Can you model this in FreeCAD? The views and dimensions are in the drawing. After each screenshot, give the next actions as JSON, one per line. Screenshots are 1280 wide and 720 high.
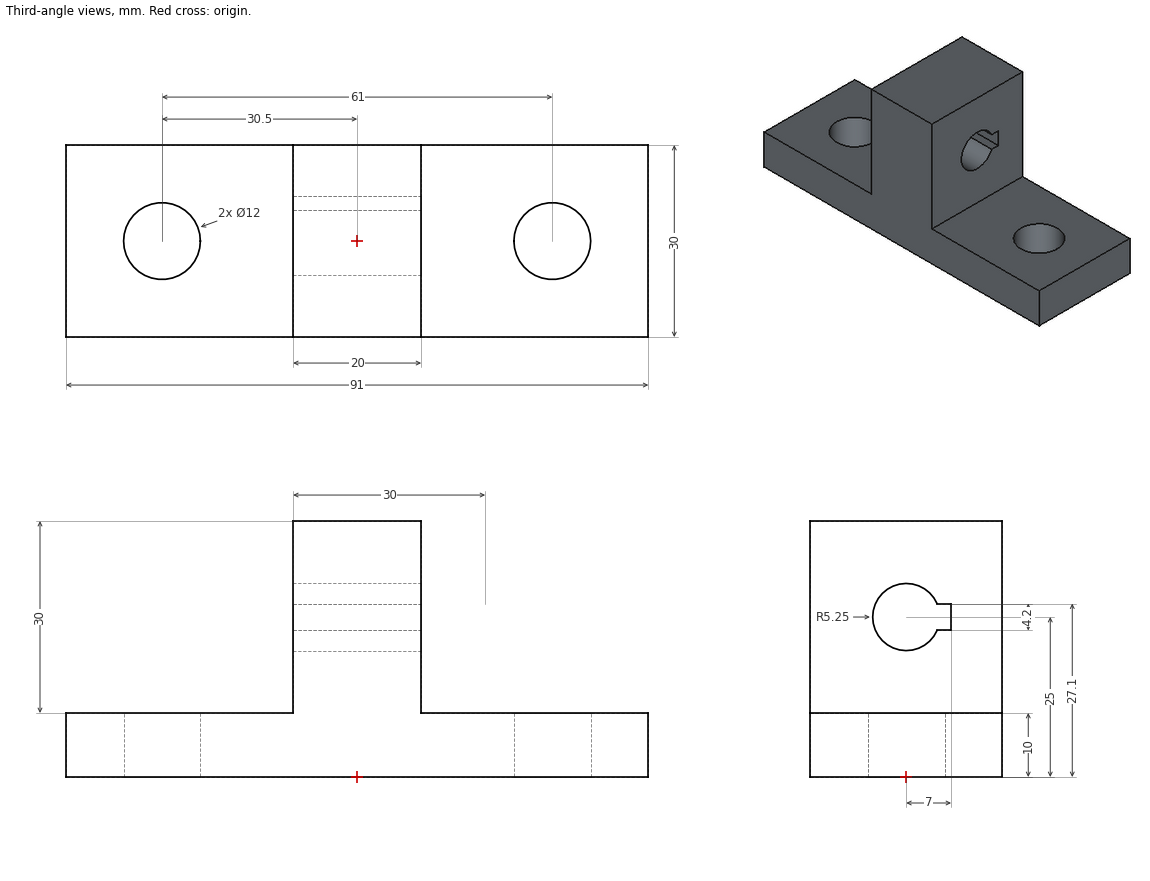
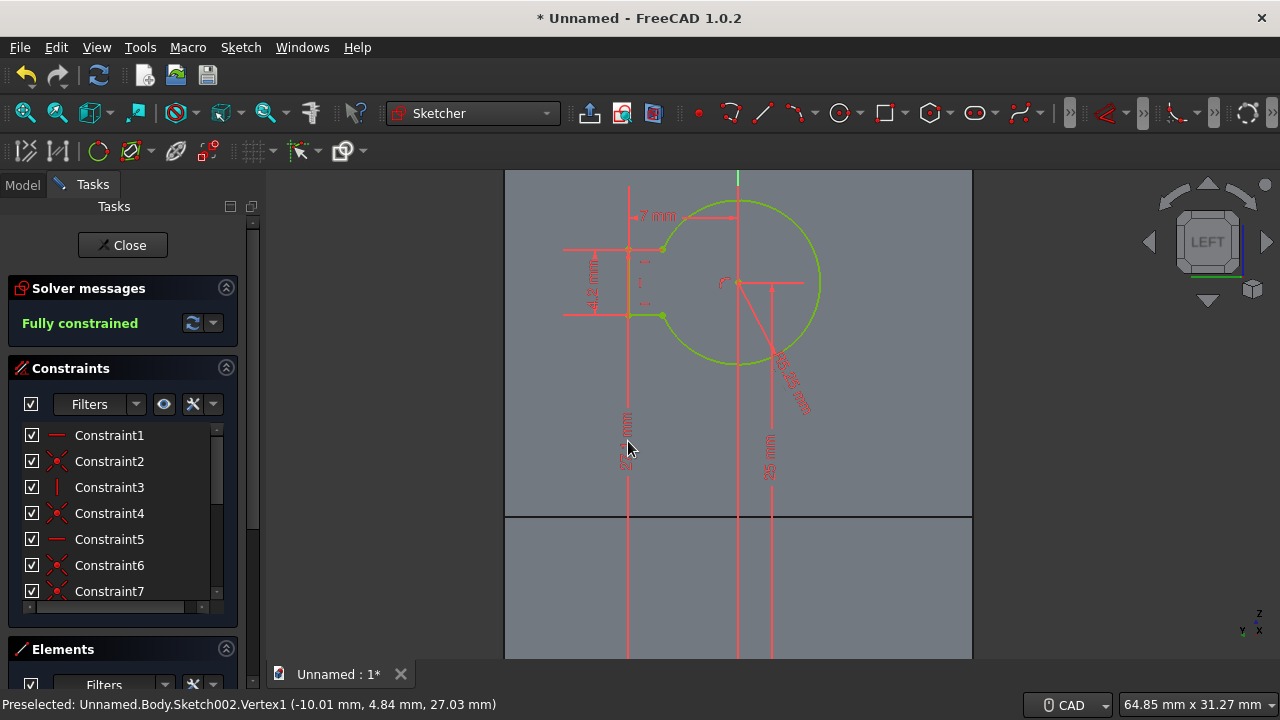
{"action": "left_click", "coordinate": [123, 245]}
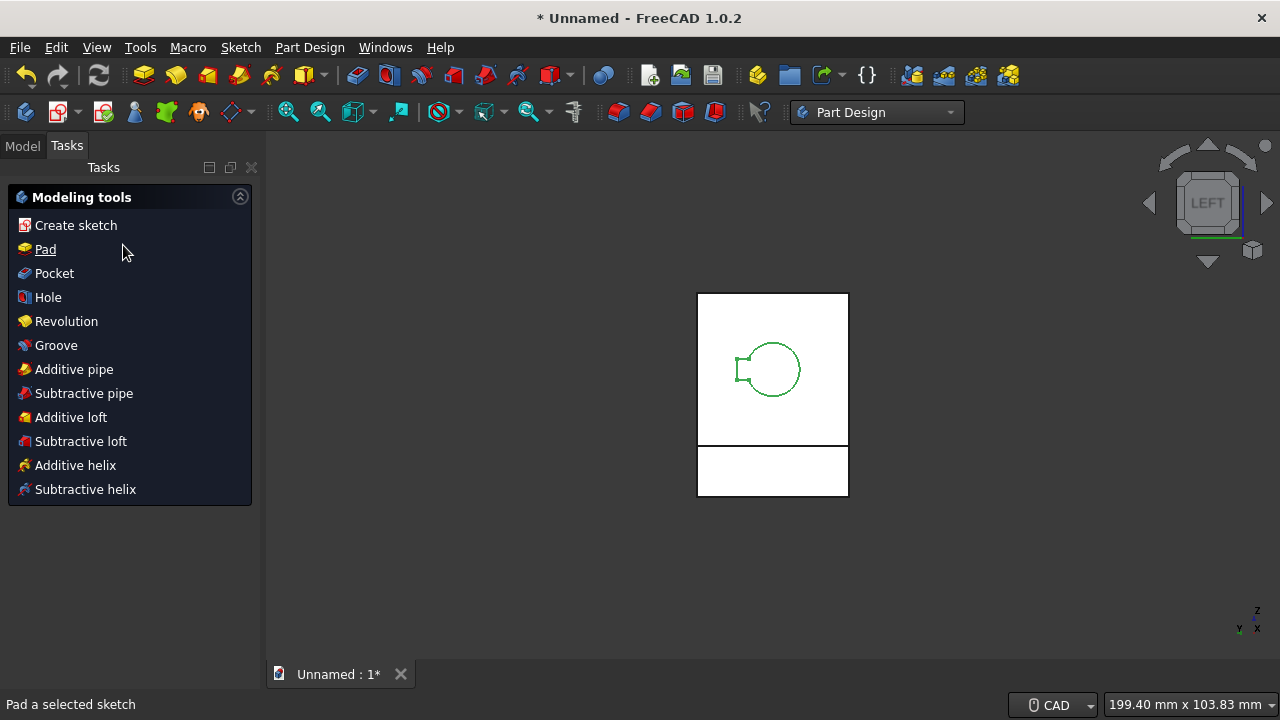
{"action": "left_click", "coordinate": [358, 76]}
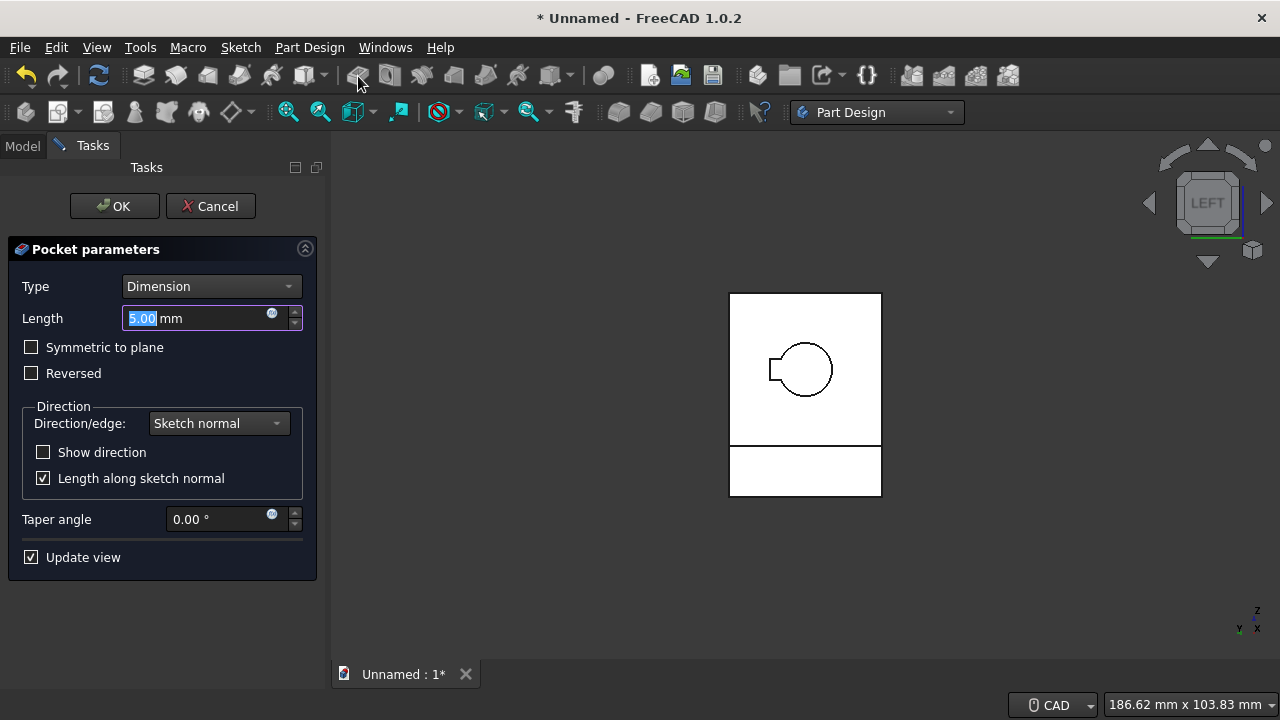
{"action": "type", "text": "30"}
{"action": "key", "text": "Tab"}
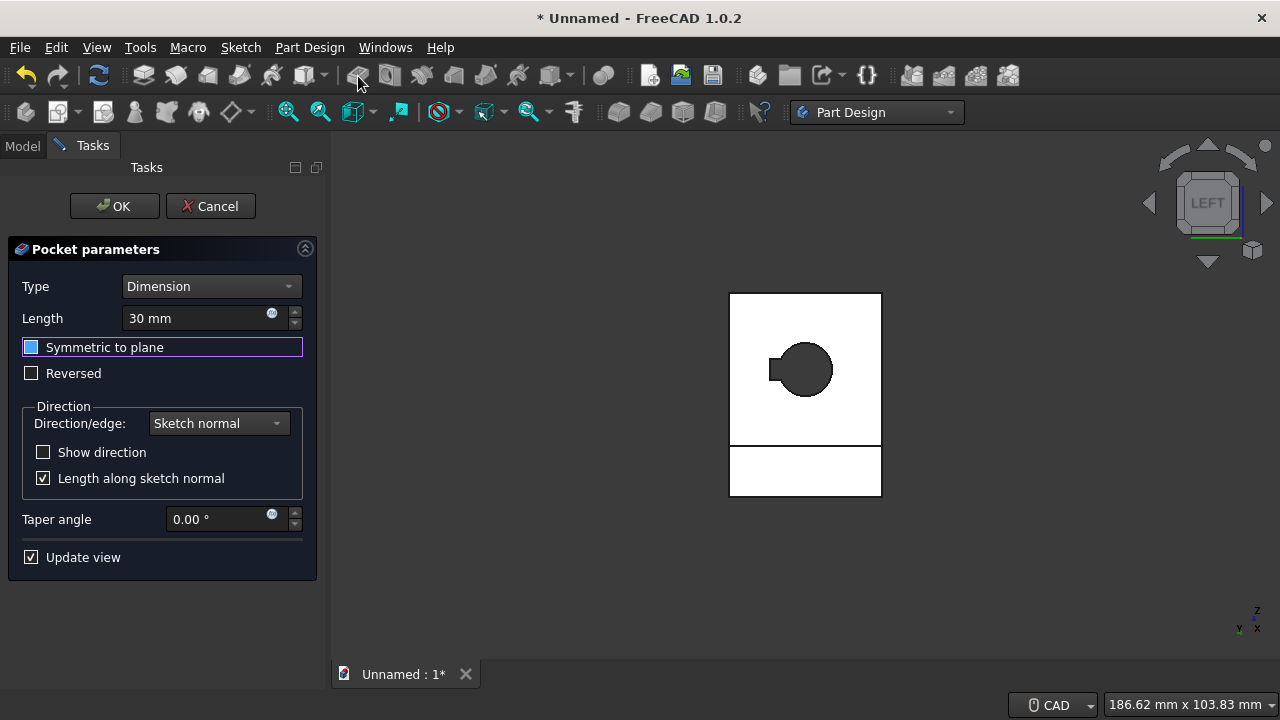
{"action": "left_click", "coordinate": [115, 206]}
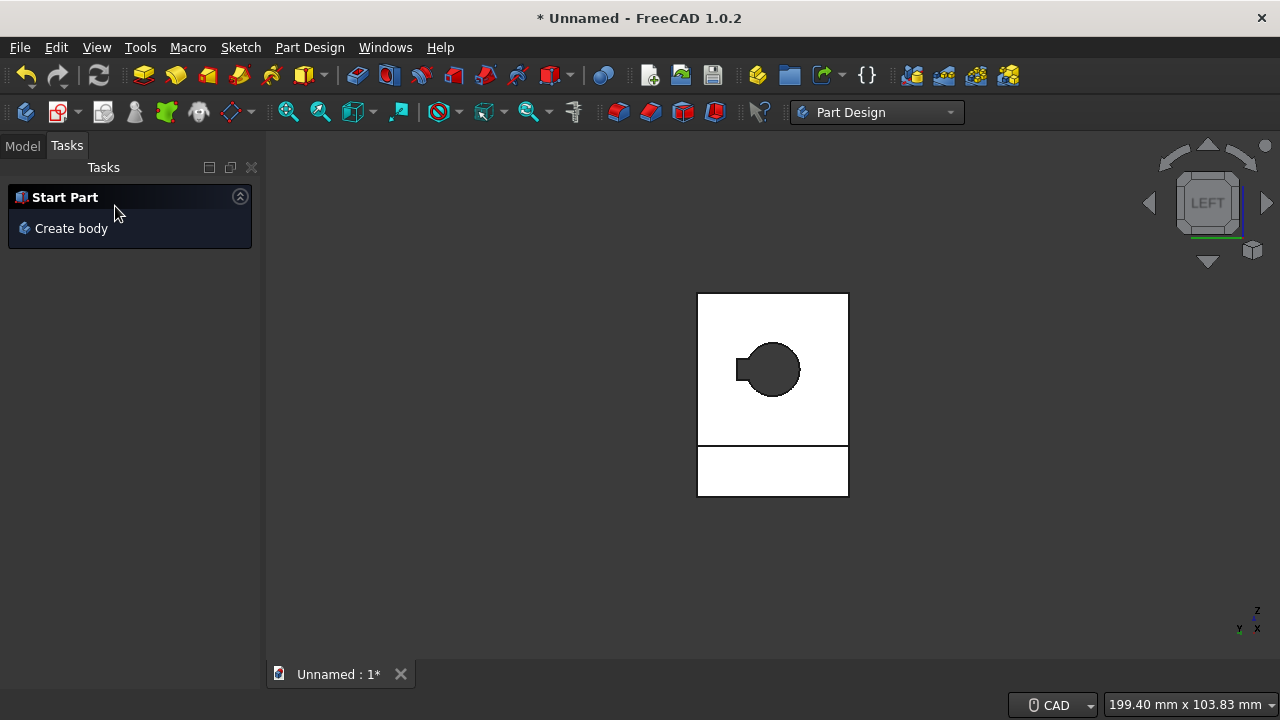
{"action": "left_click", "coordinate": [290, 112]}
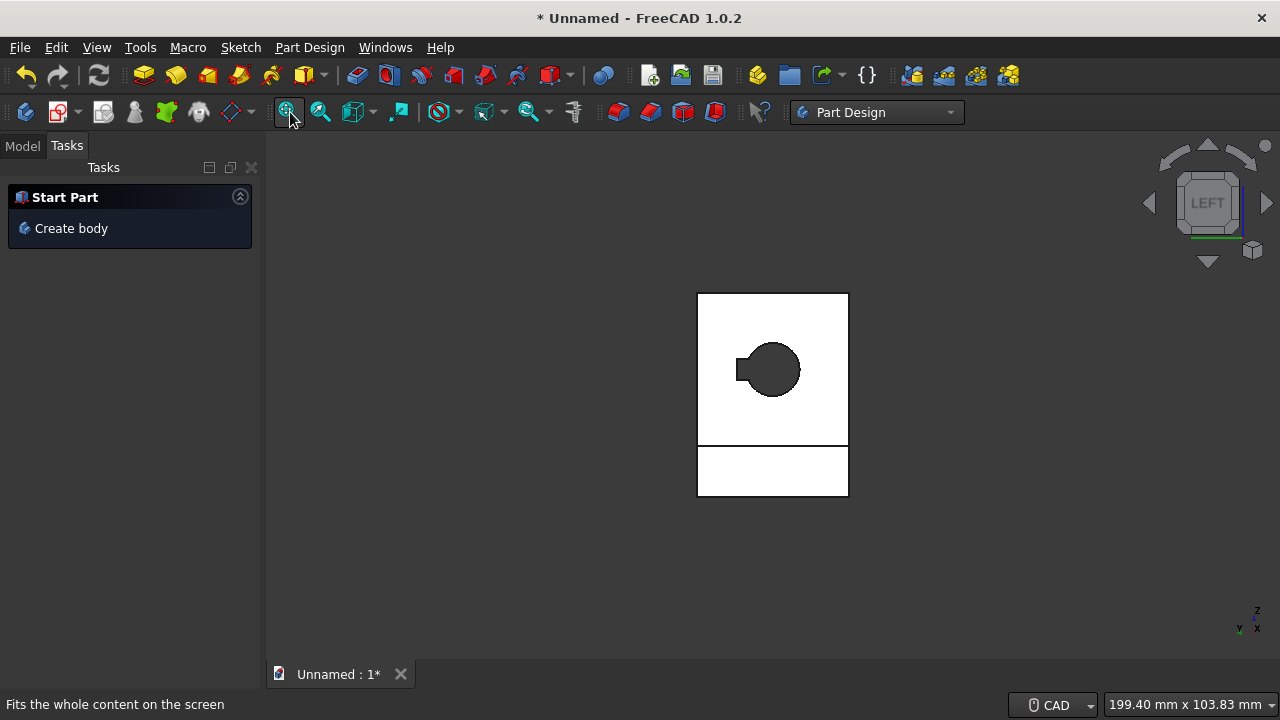
{"action": "key", "text": "0"}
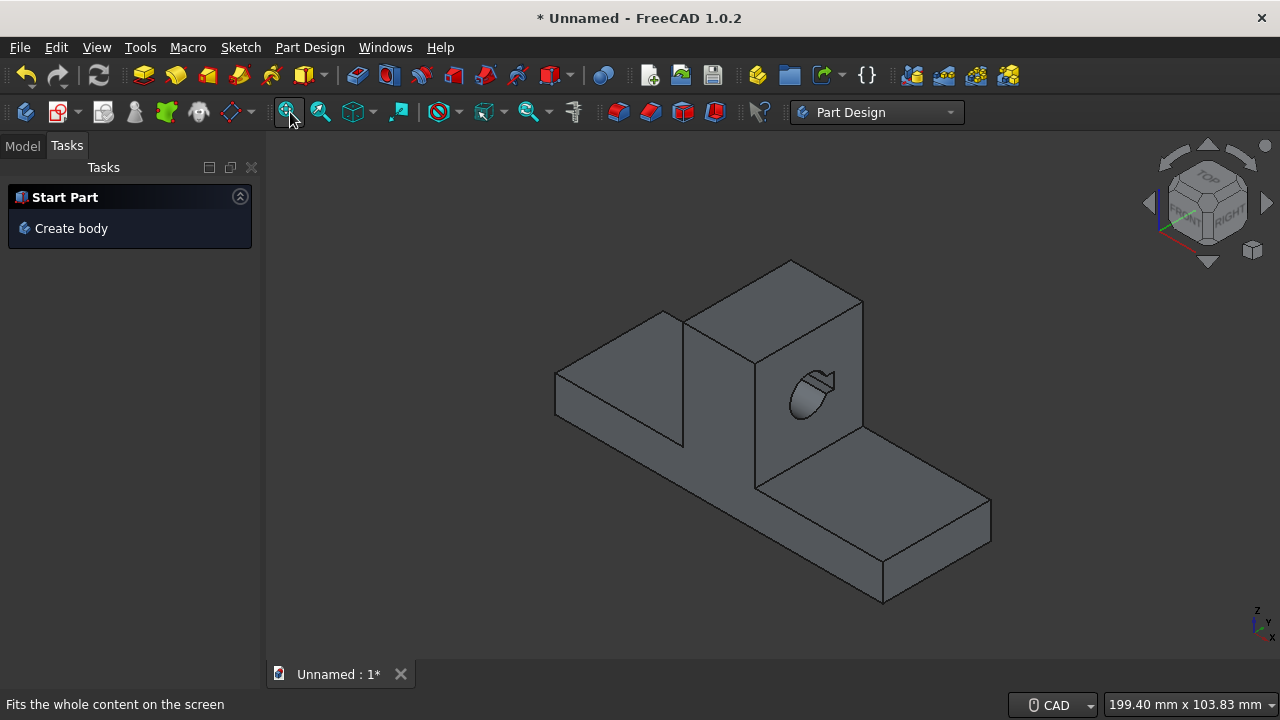
{"action": "left_click", "coordinate": [873, 493]}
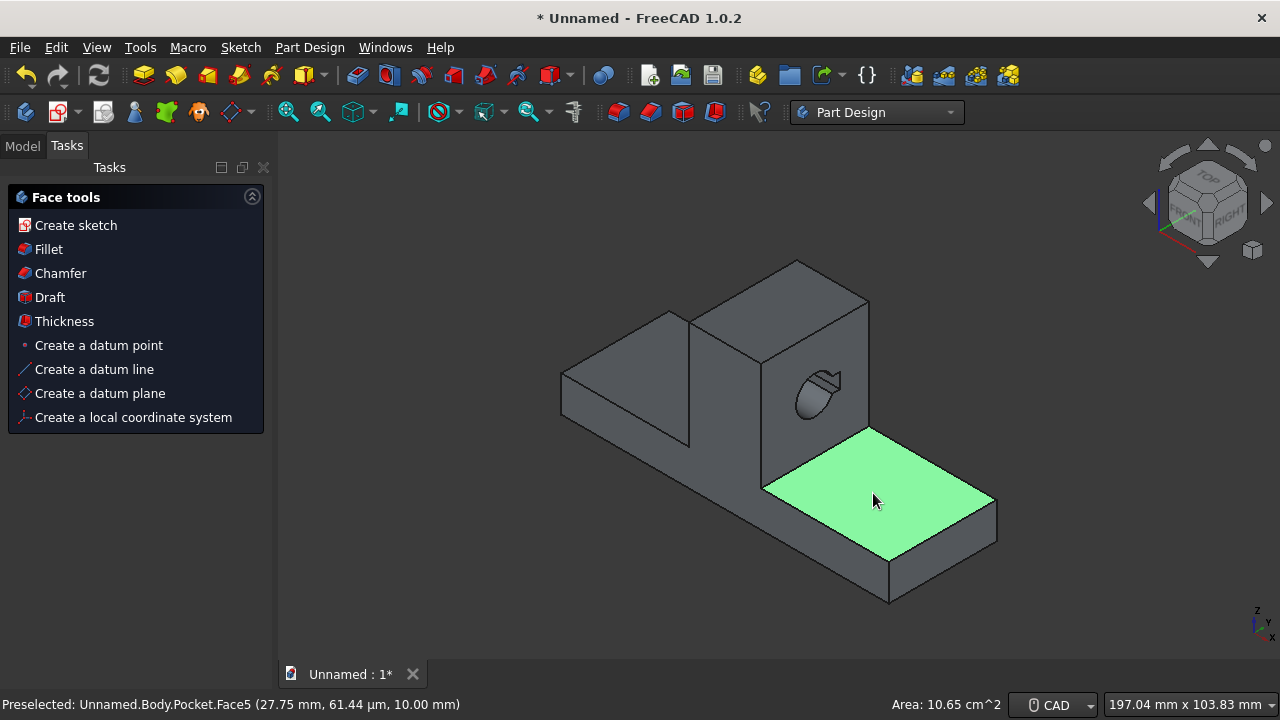
{"action": "left_click", "coordinate": [58, 112]}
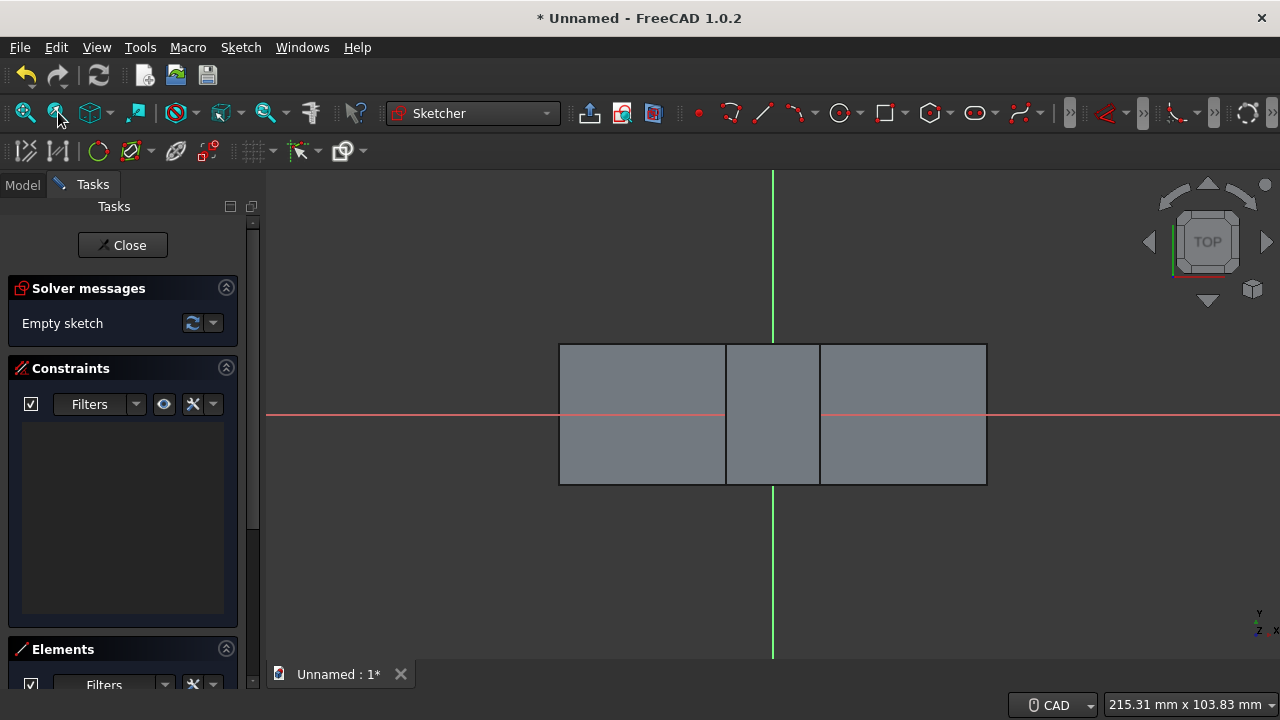
{"action": "scroll", "coordinate": [856, 415], "scroll_direction": "up", "scroll_amount": 3}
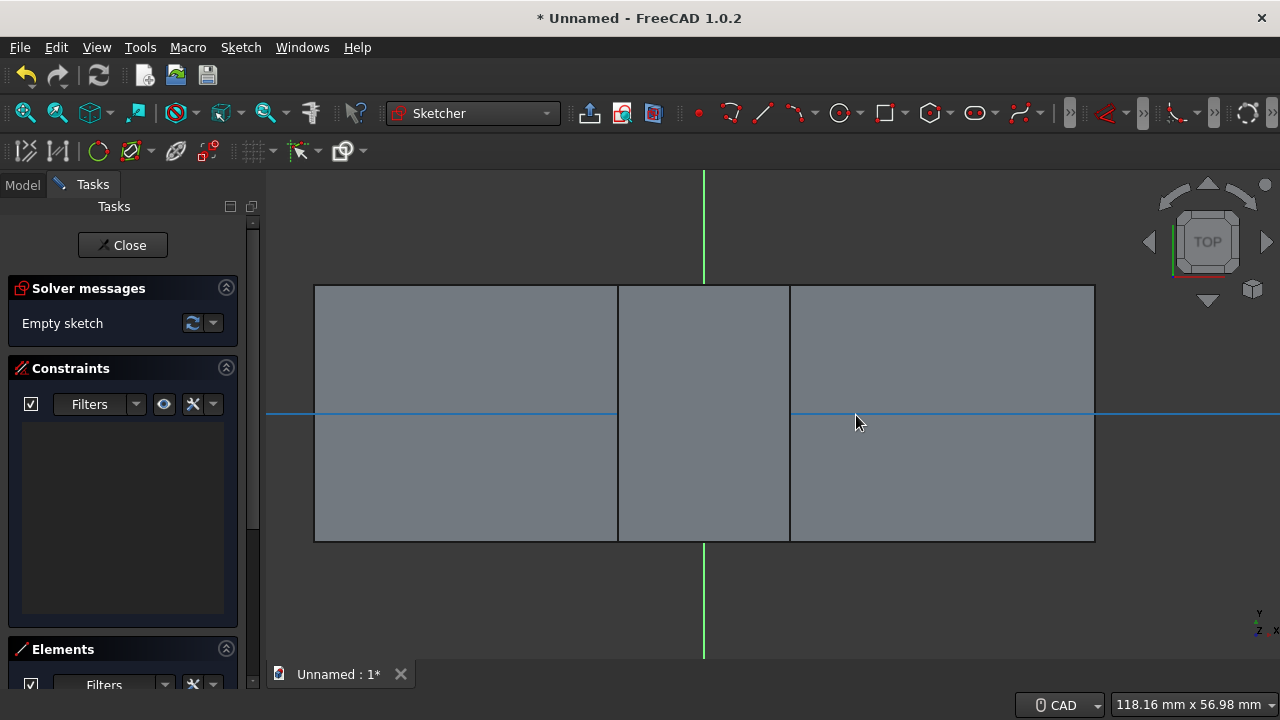
{"action": "left_click", "coordinate": [840, 114]}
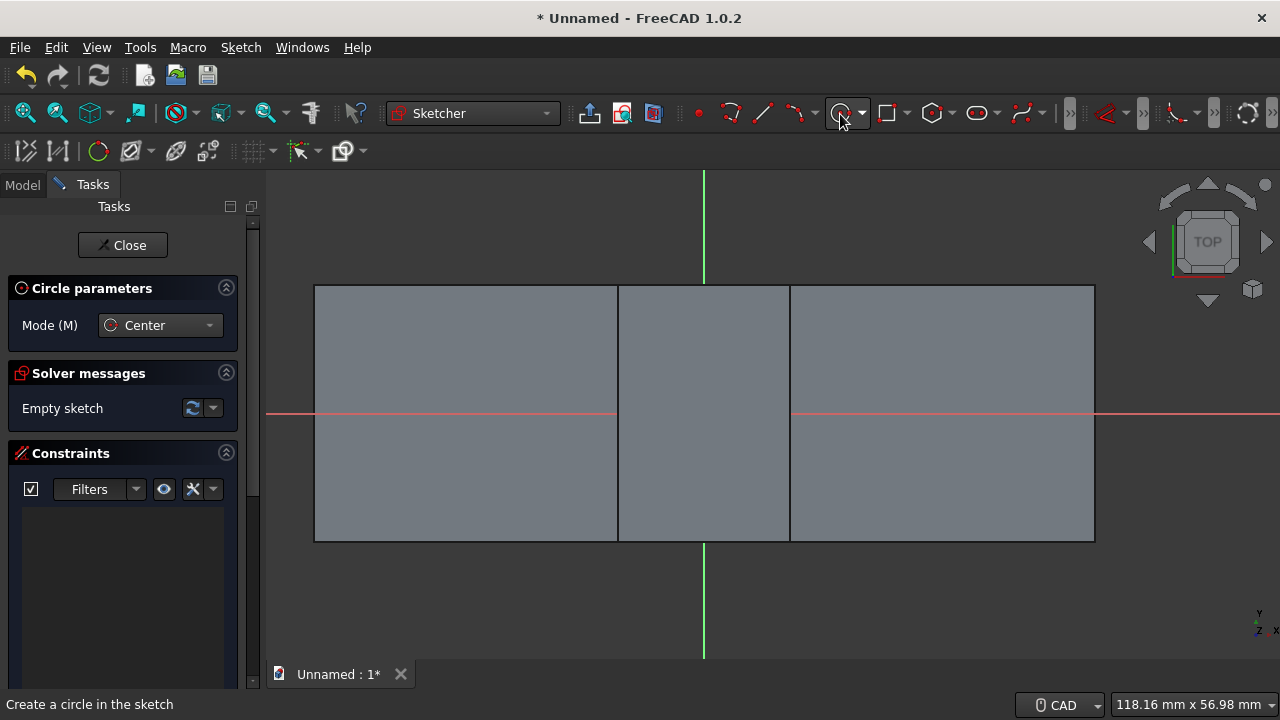
{"action": "left_click", "coordinate": [443, 414]}
{"action": "left_click", "coordinate": [479, 377]}